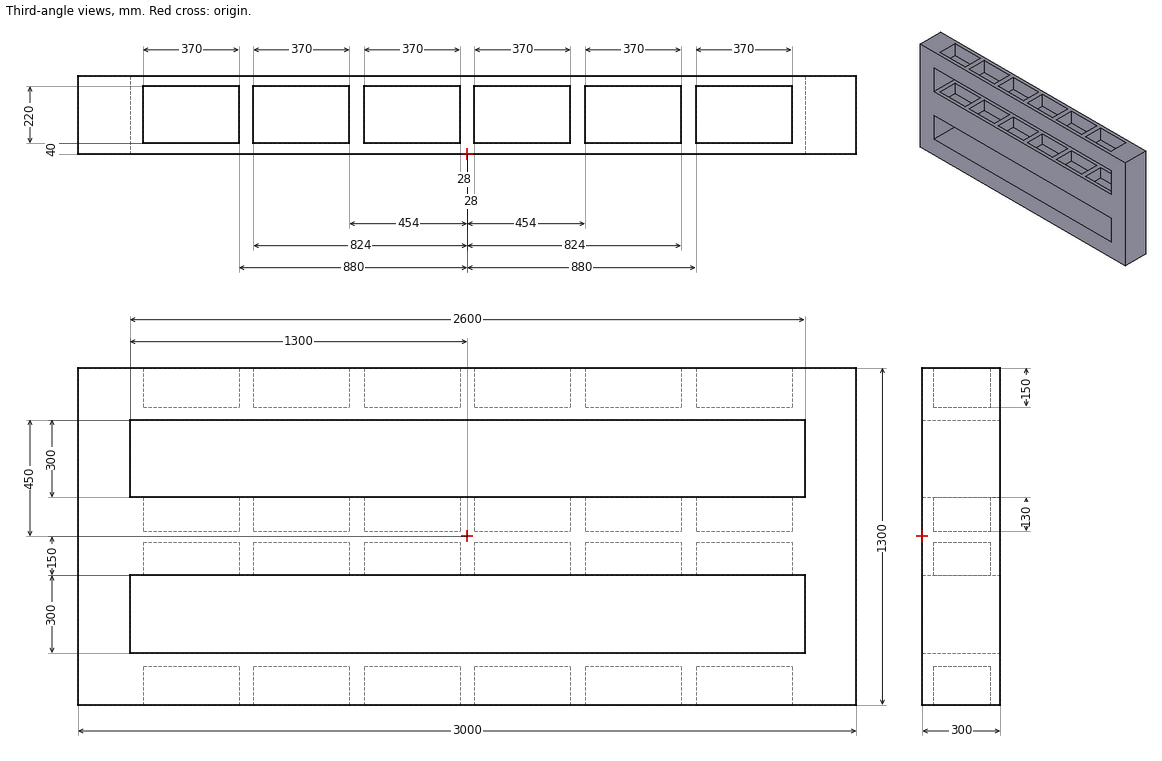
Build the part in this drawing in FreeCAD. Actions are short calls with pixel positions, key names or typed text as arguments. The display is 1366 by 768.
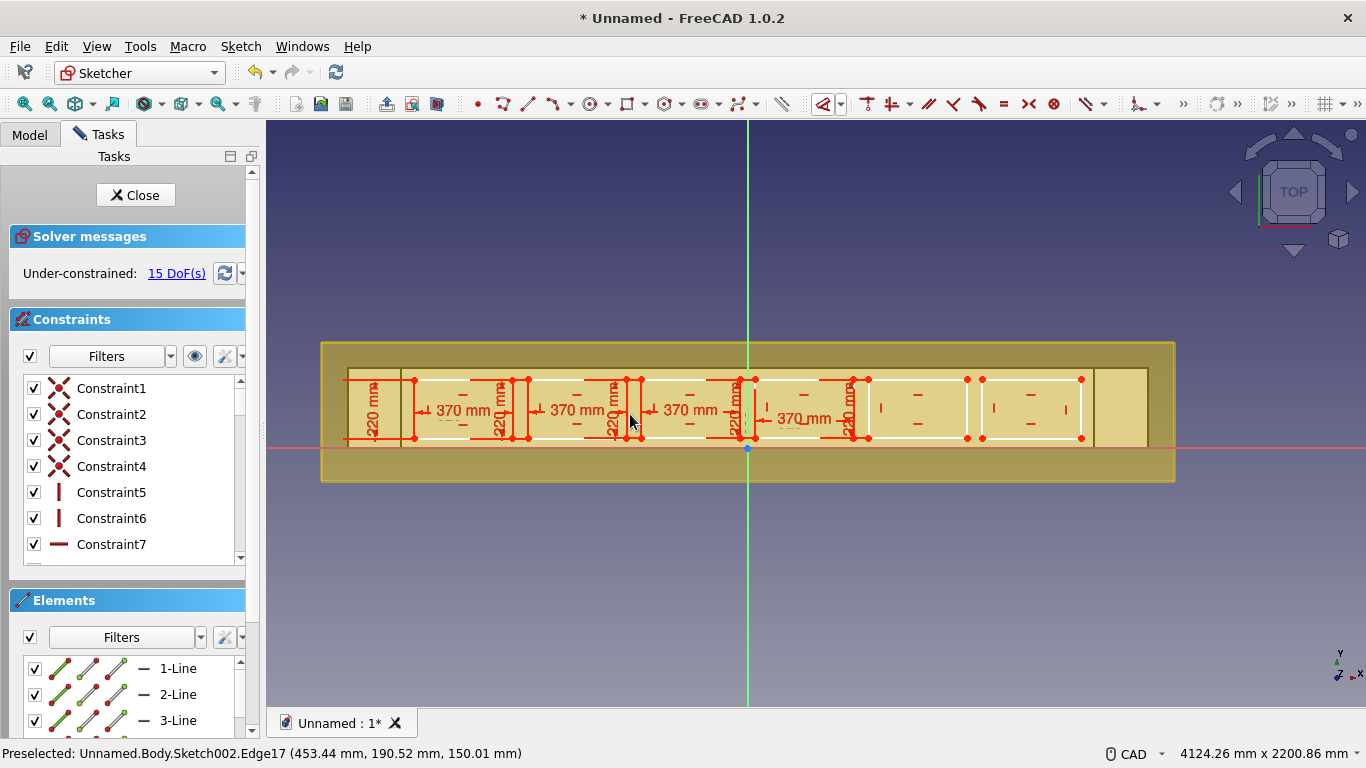
scroll(898, 438, up, 2)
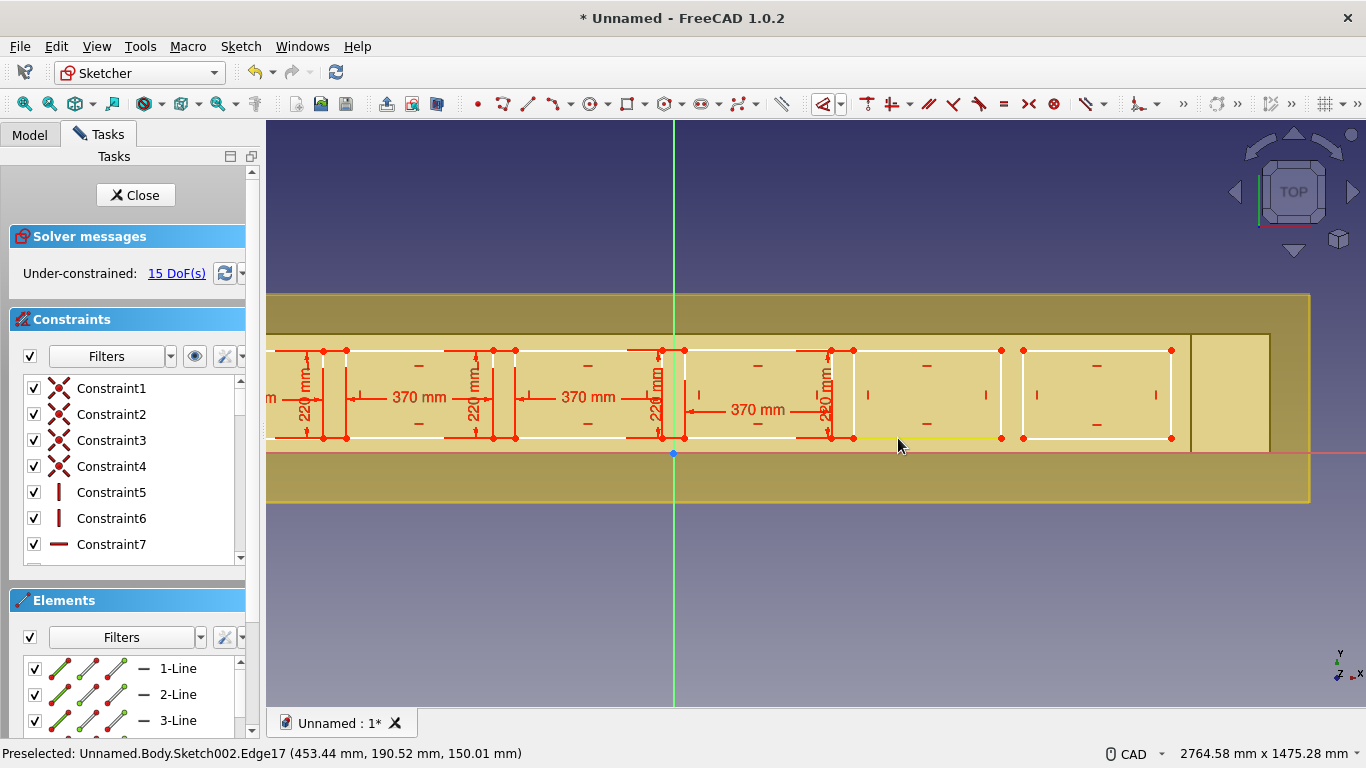
click(898, 438)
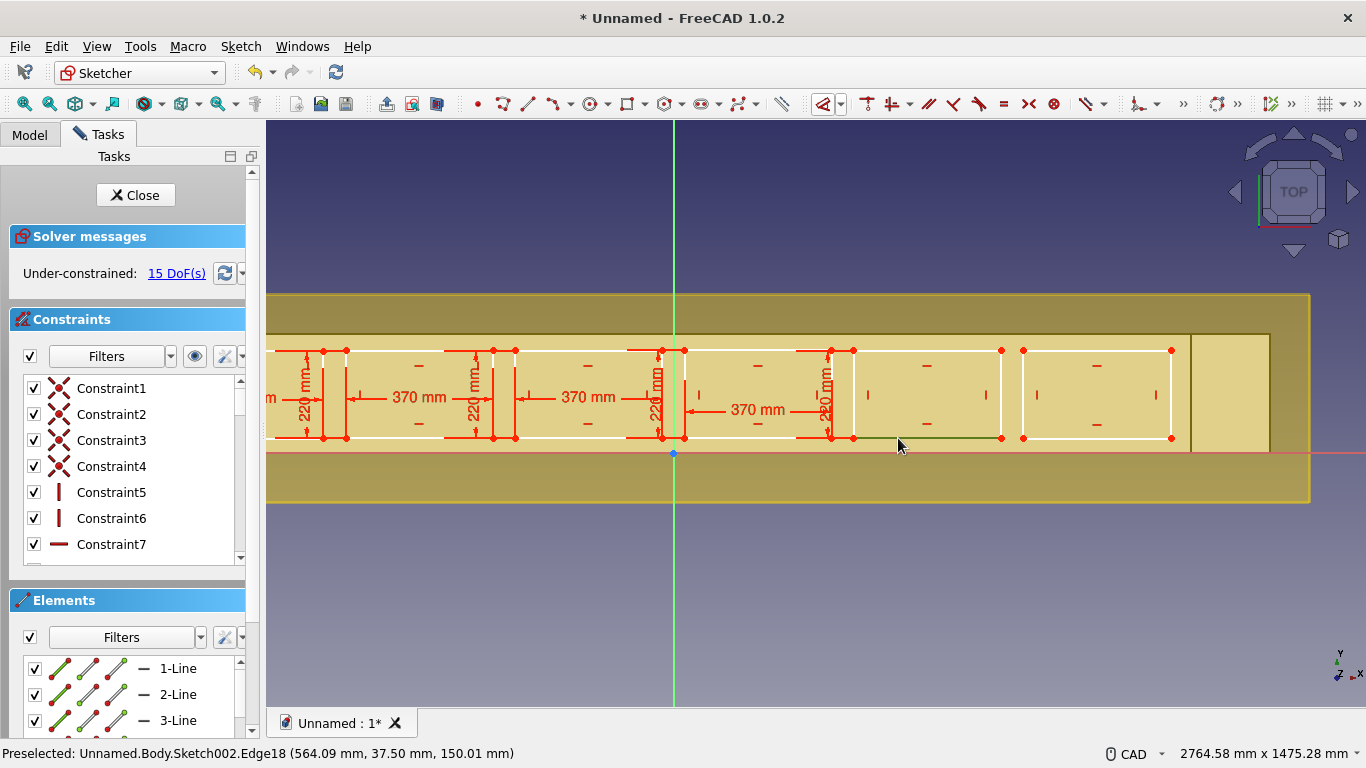
key(l)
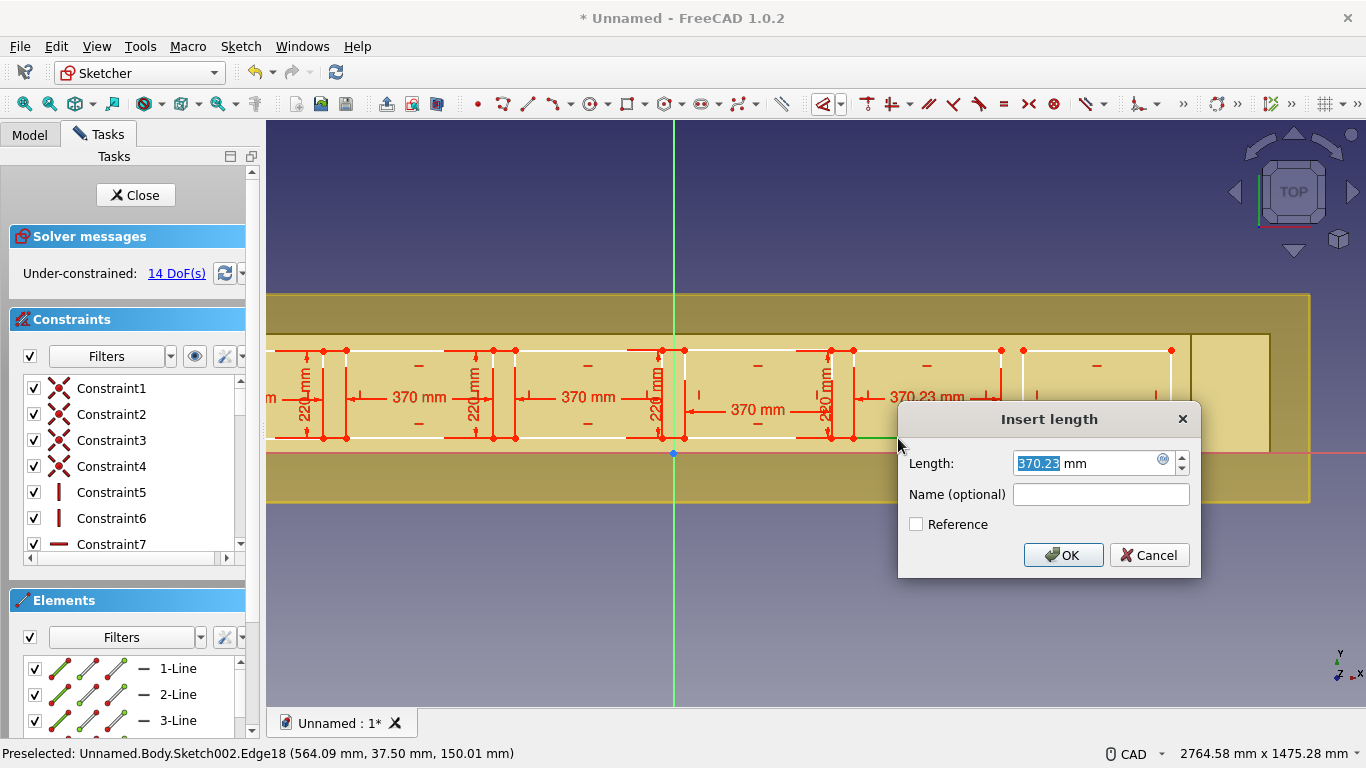
text(370)
key(Return)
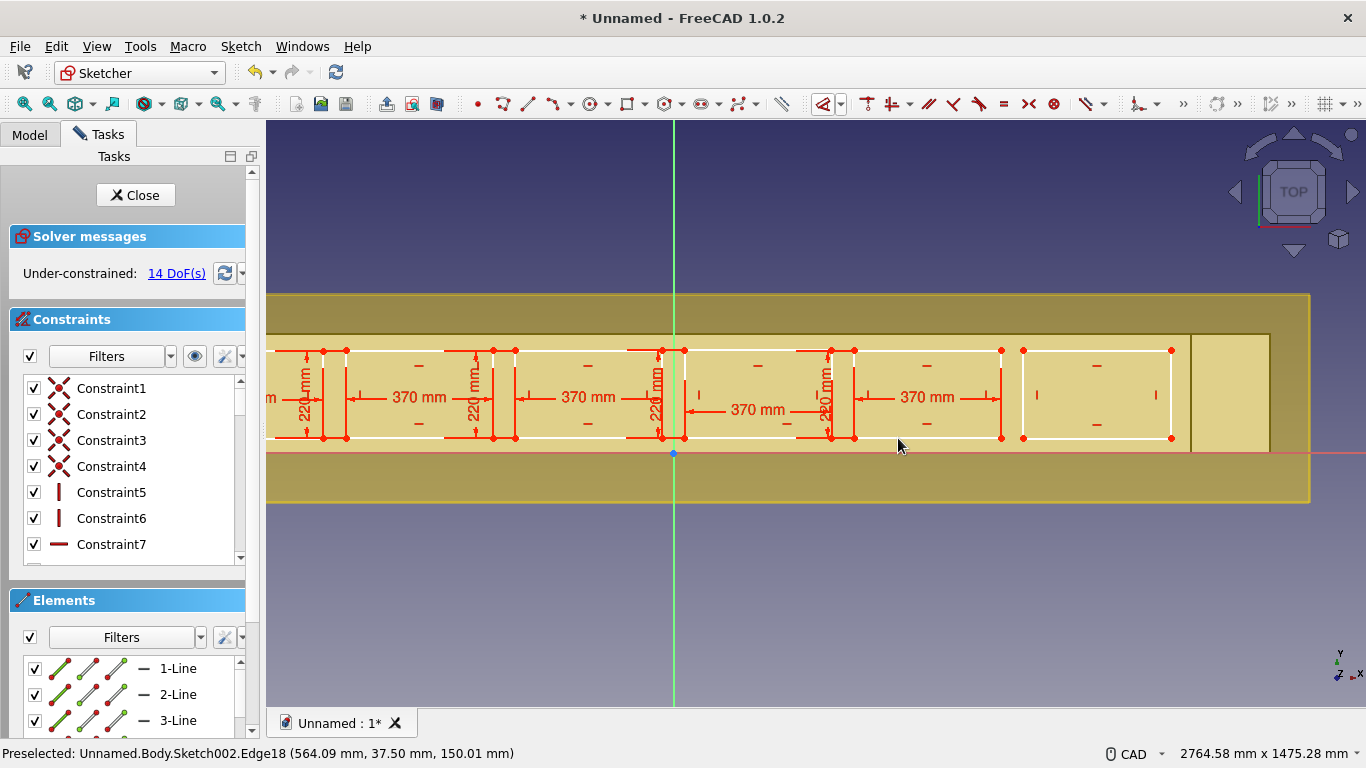
click(1023, 377)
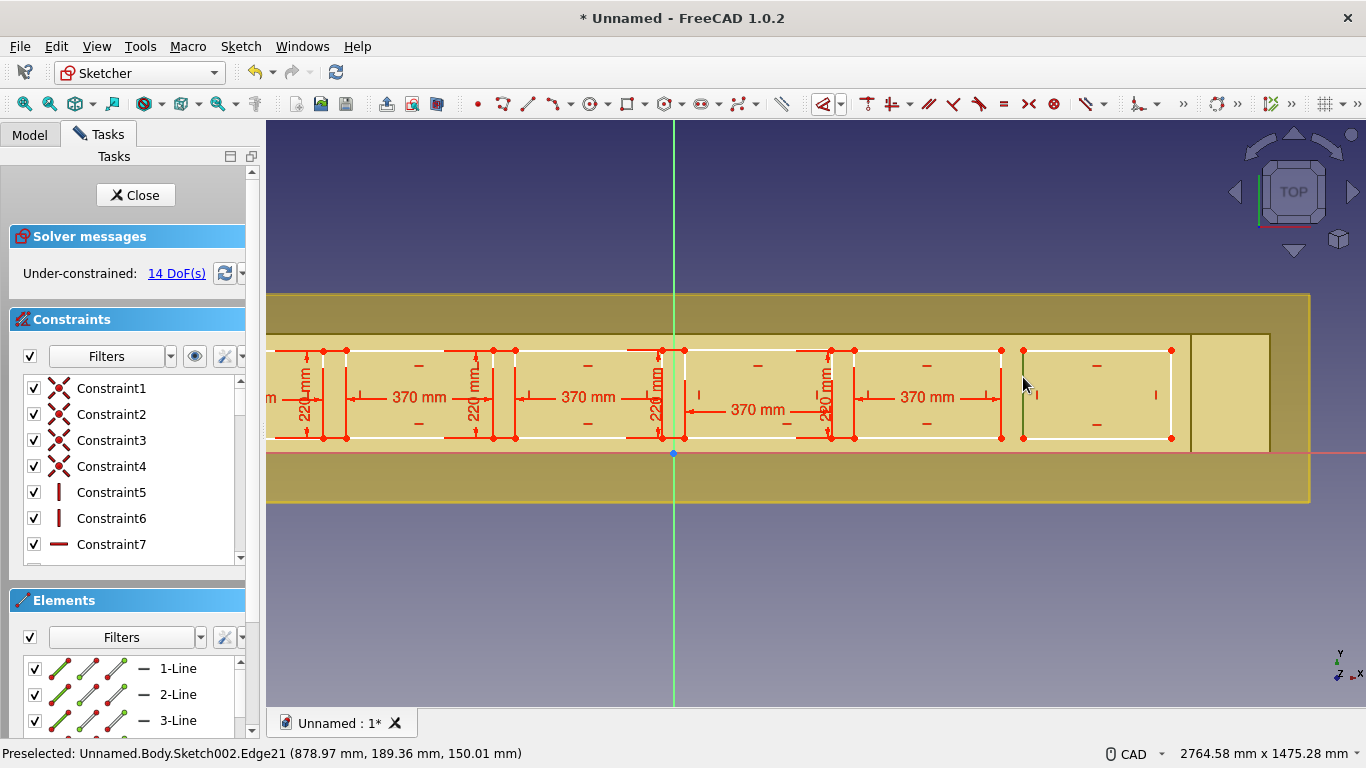
key(i)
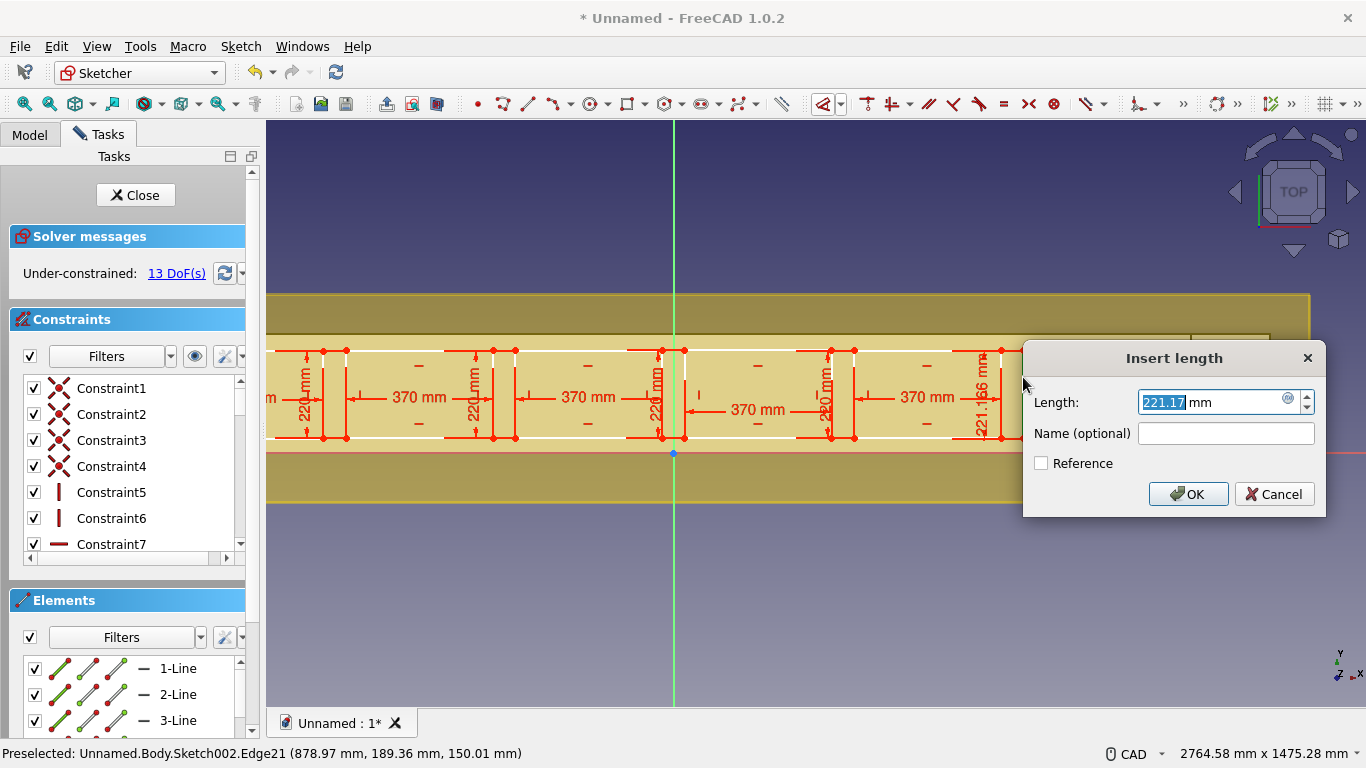
text(220)
key(Return)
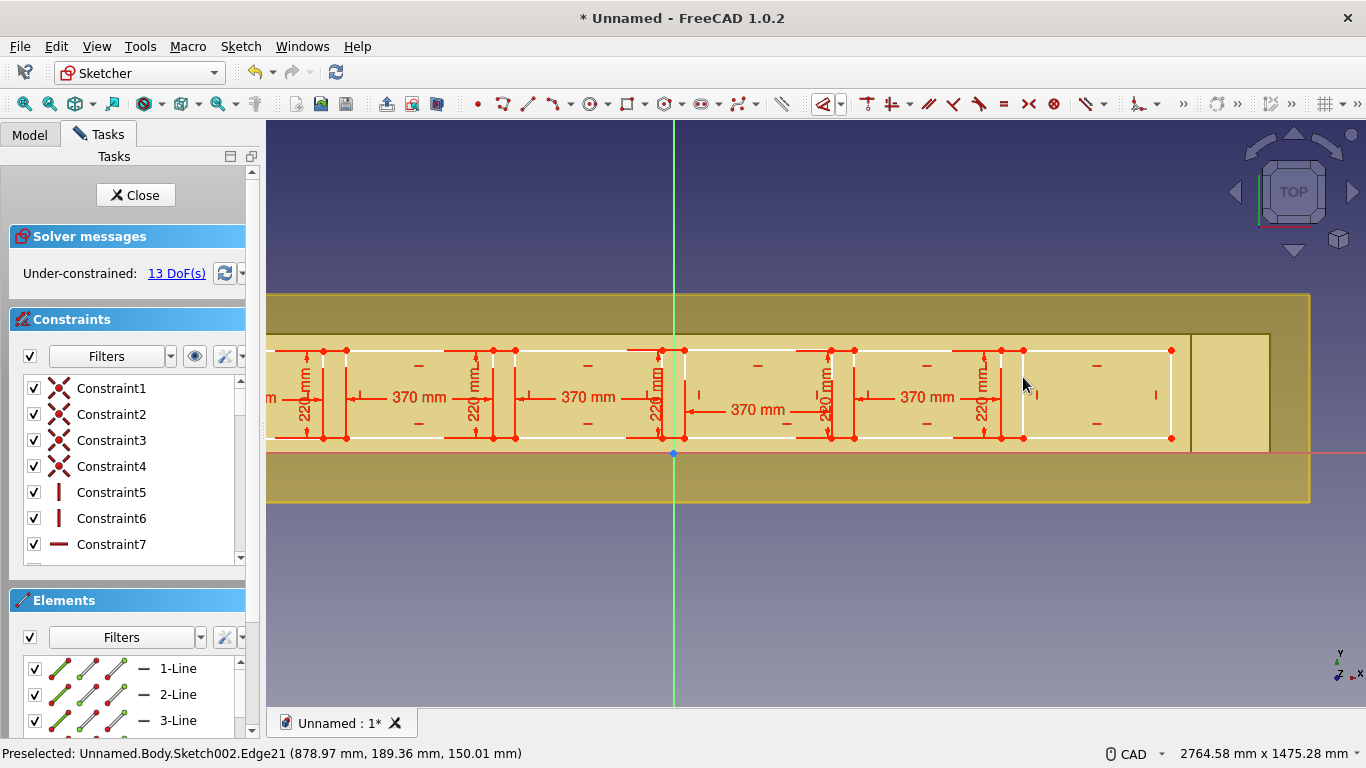
click(1068, 438)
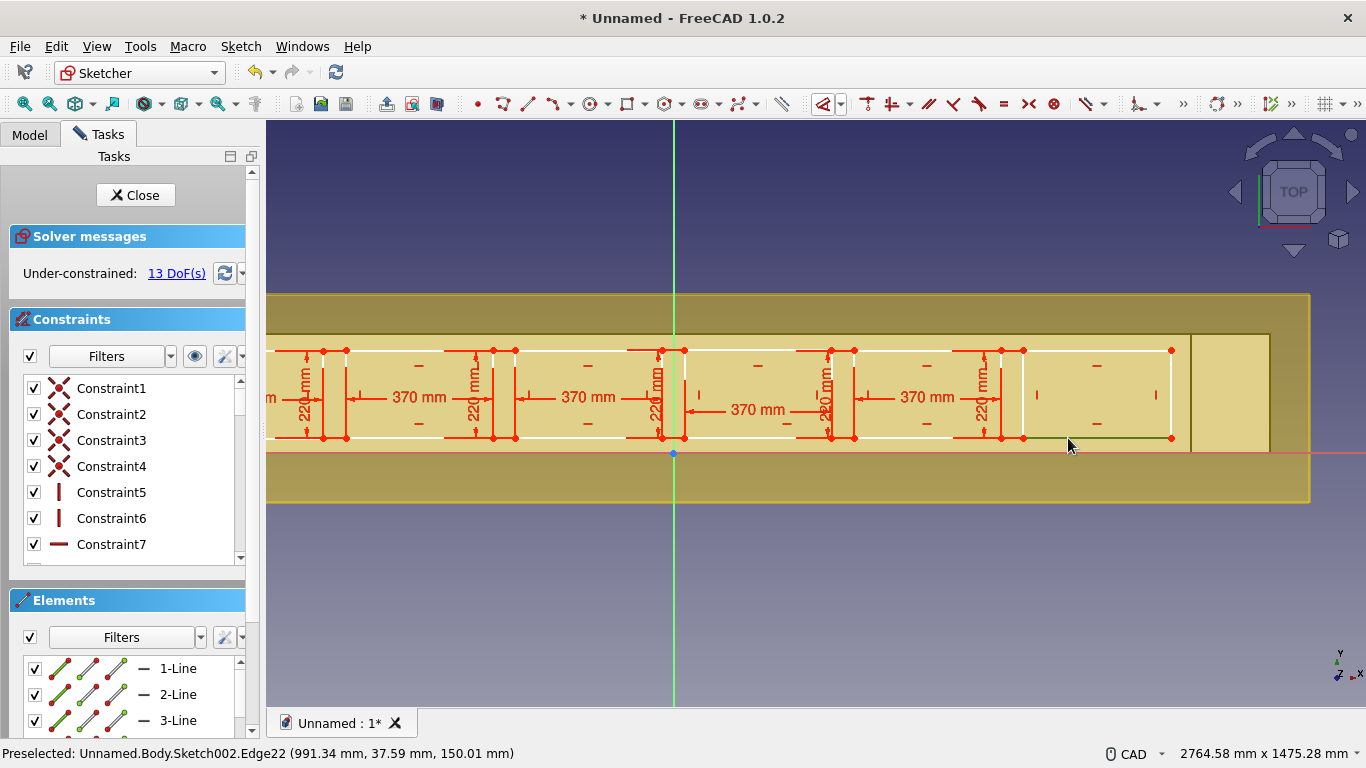
key(l)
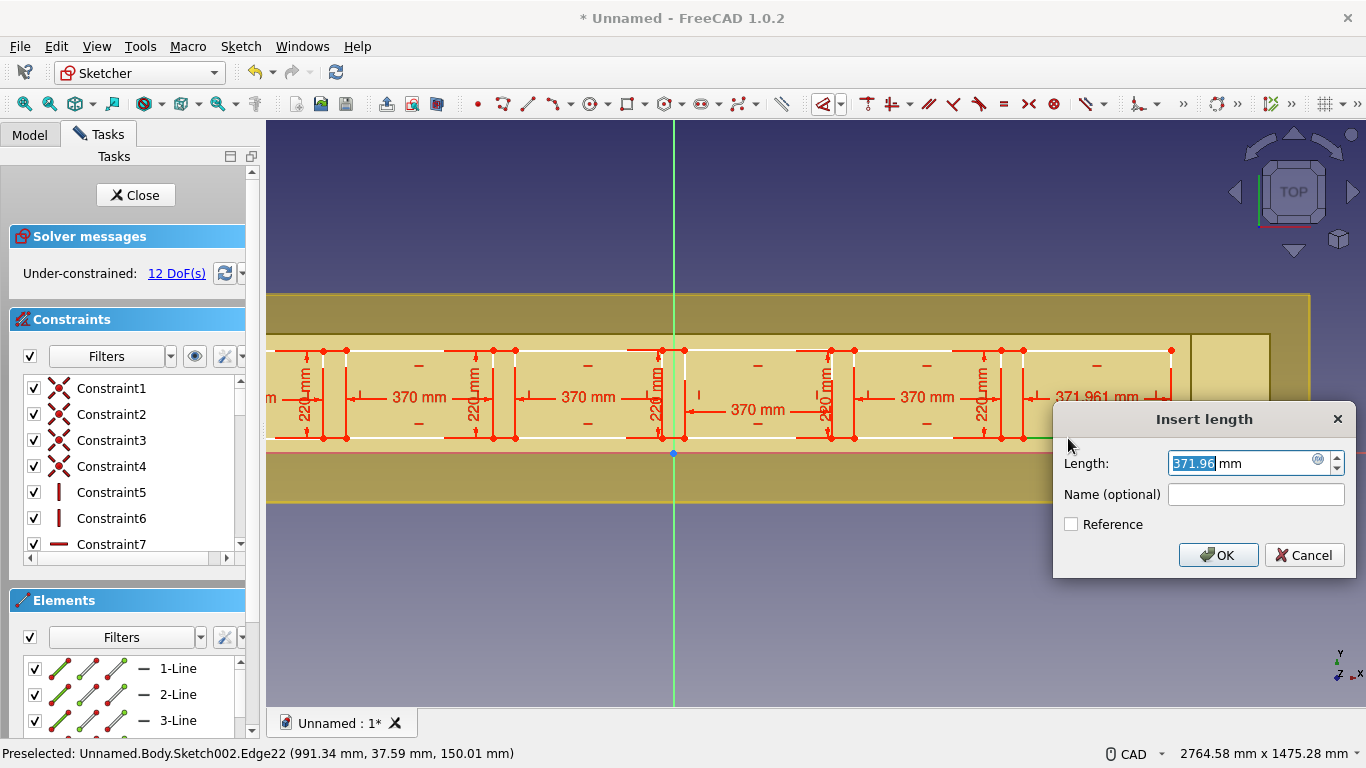
text(370)
key(Return)